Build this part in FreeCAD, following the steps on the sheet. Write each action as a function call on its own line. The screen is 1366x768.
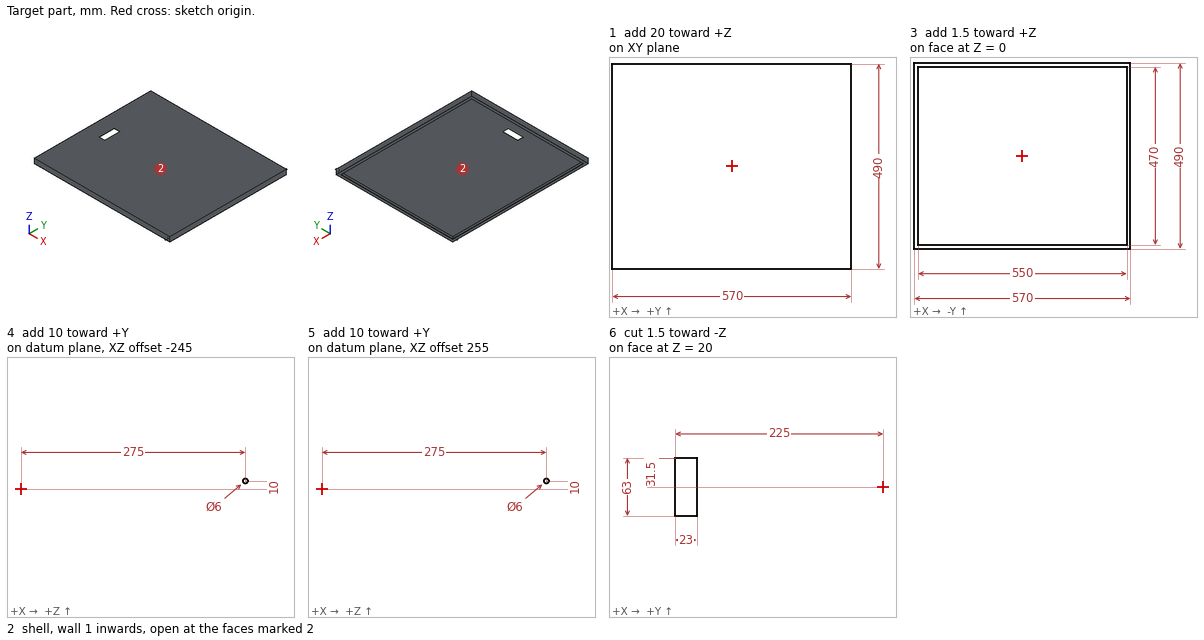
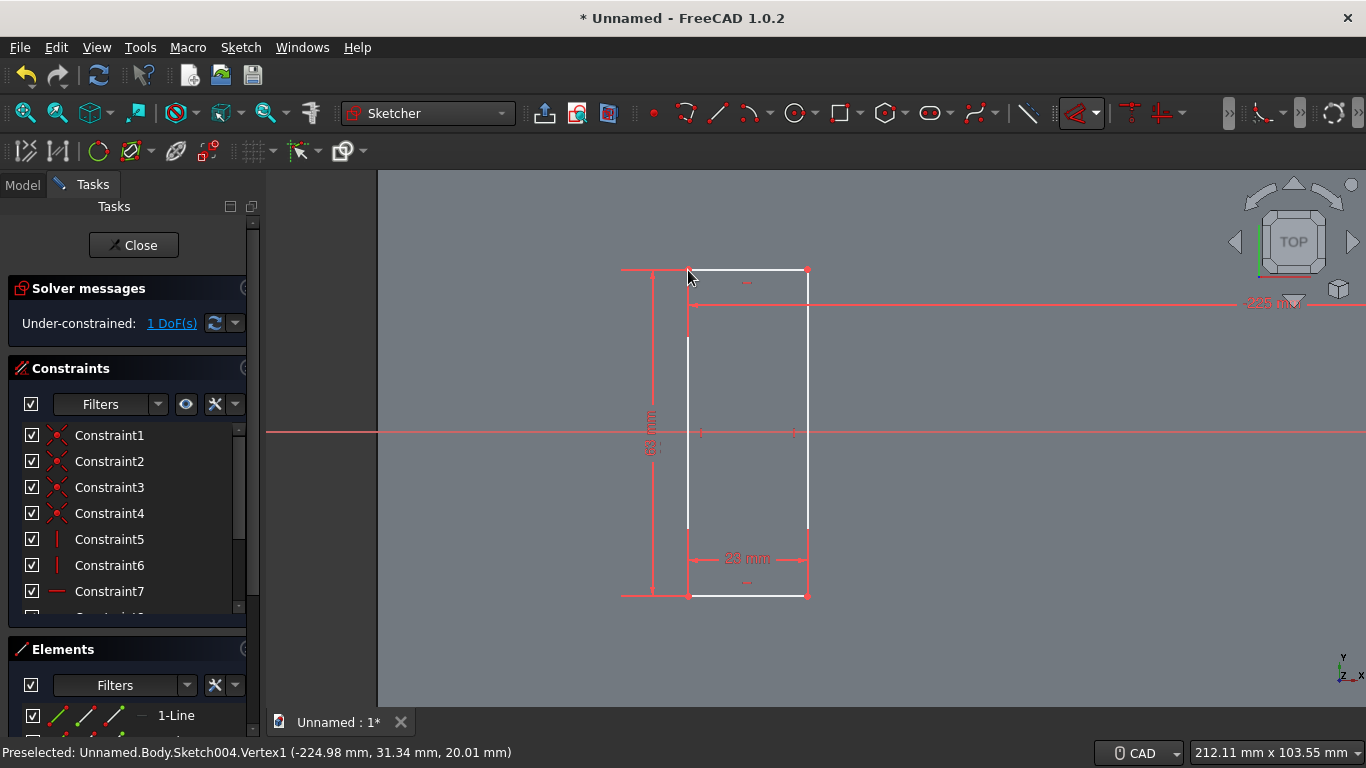
click(688, 270)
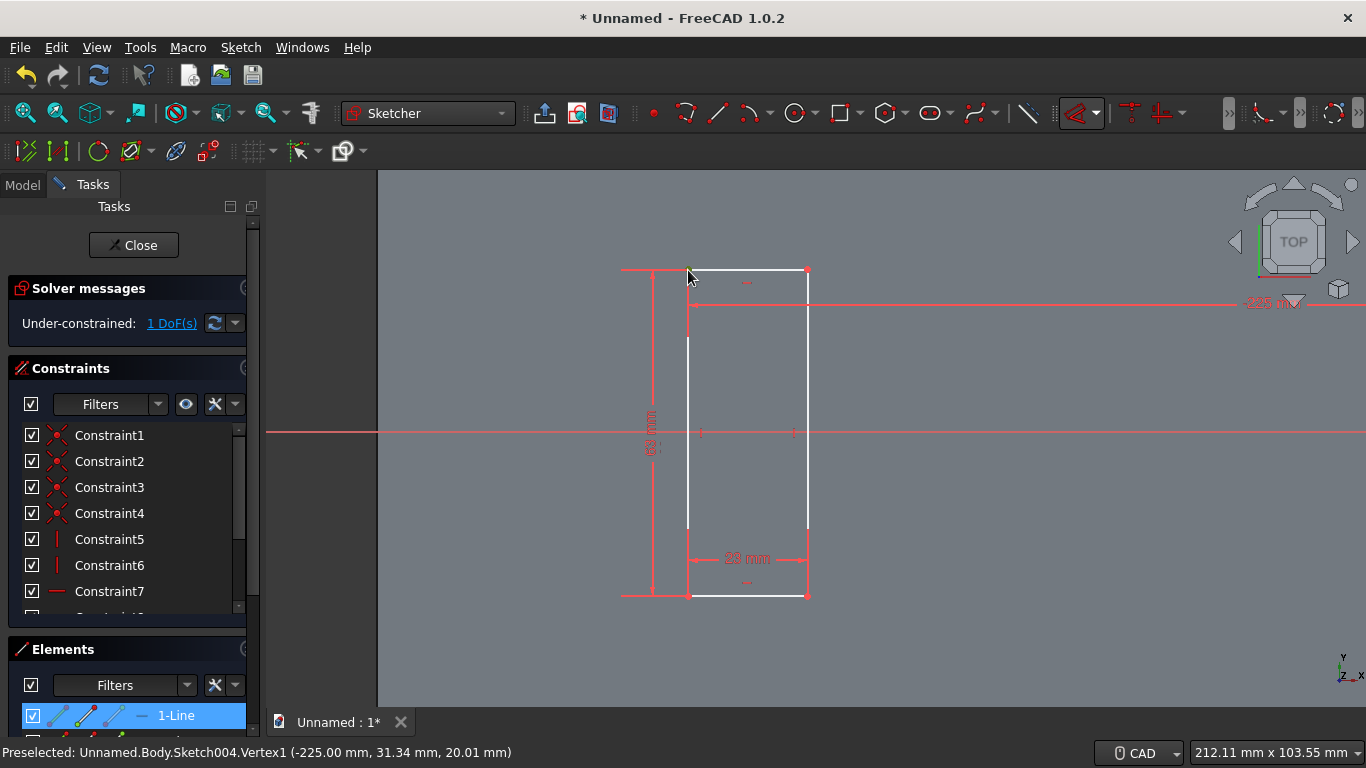
click(1098, 114)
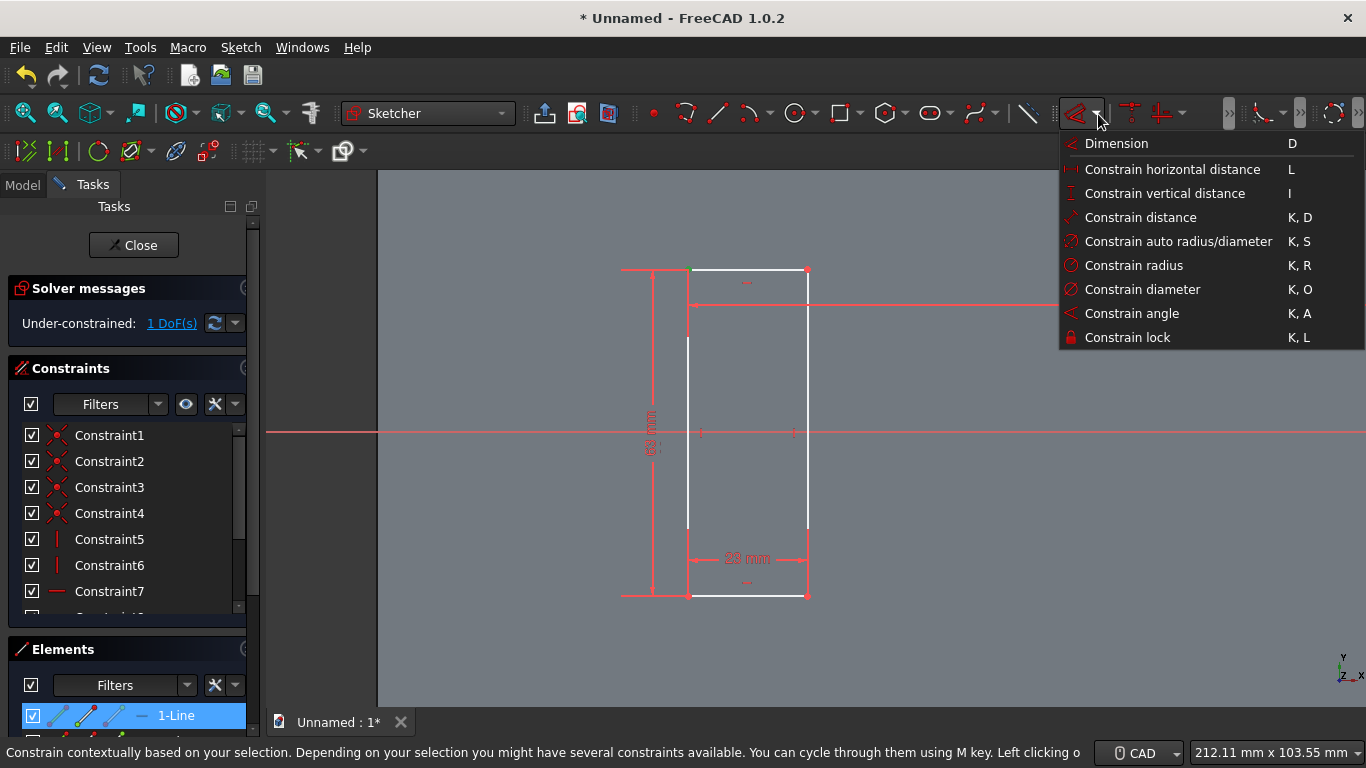
click(1212, 193)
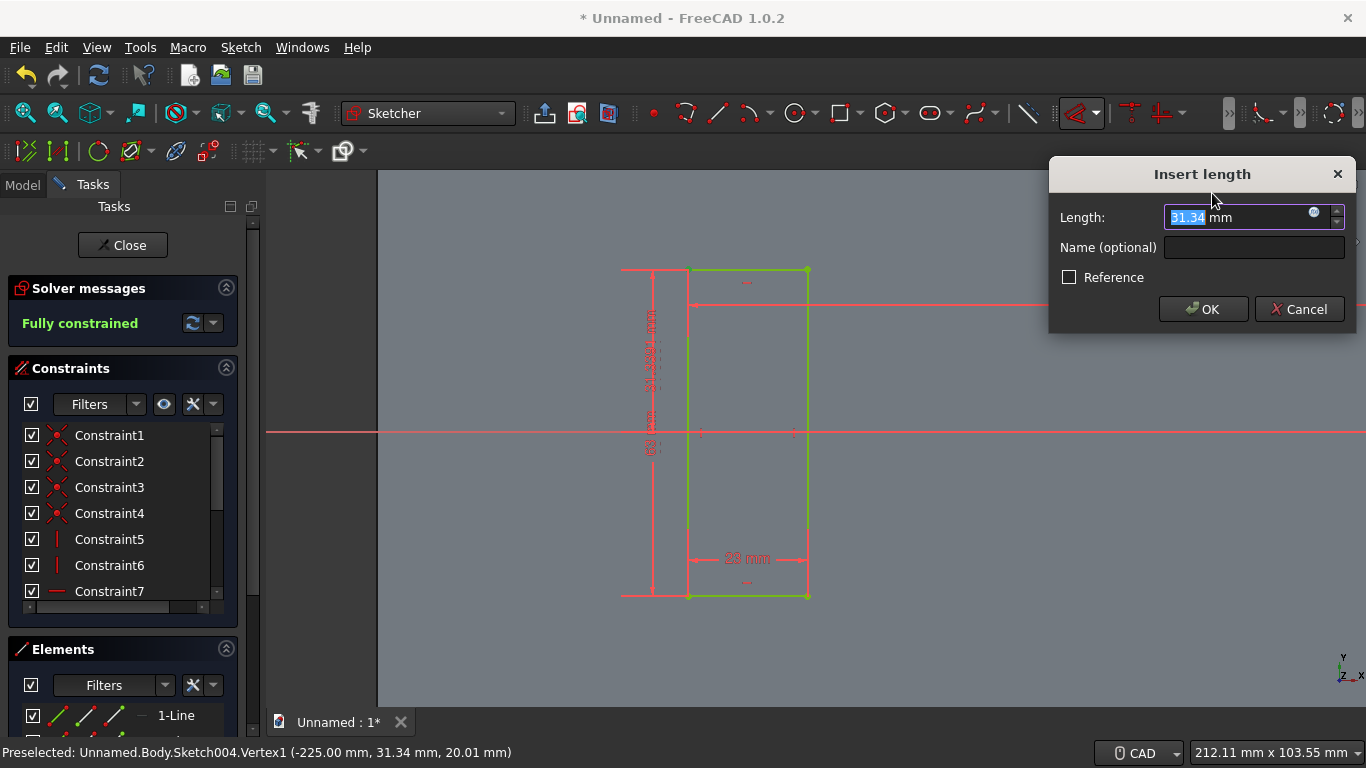
text(31.5)
key(Return)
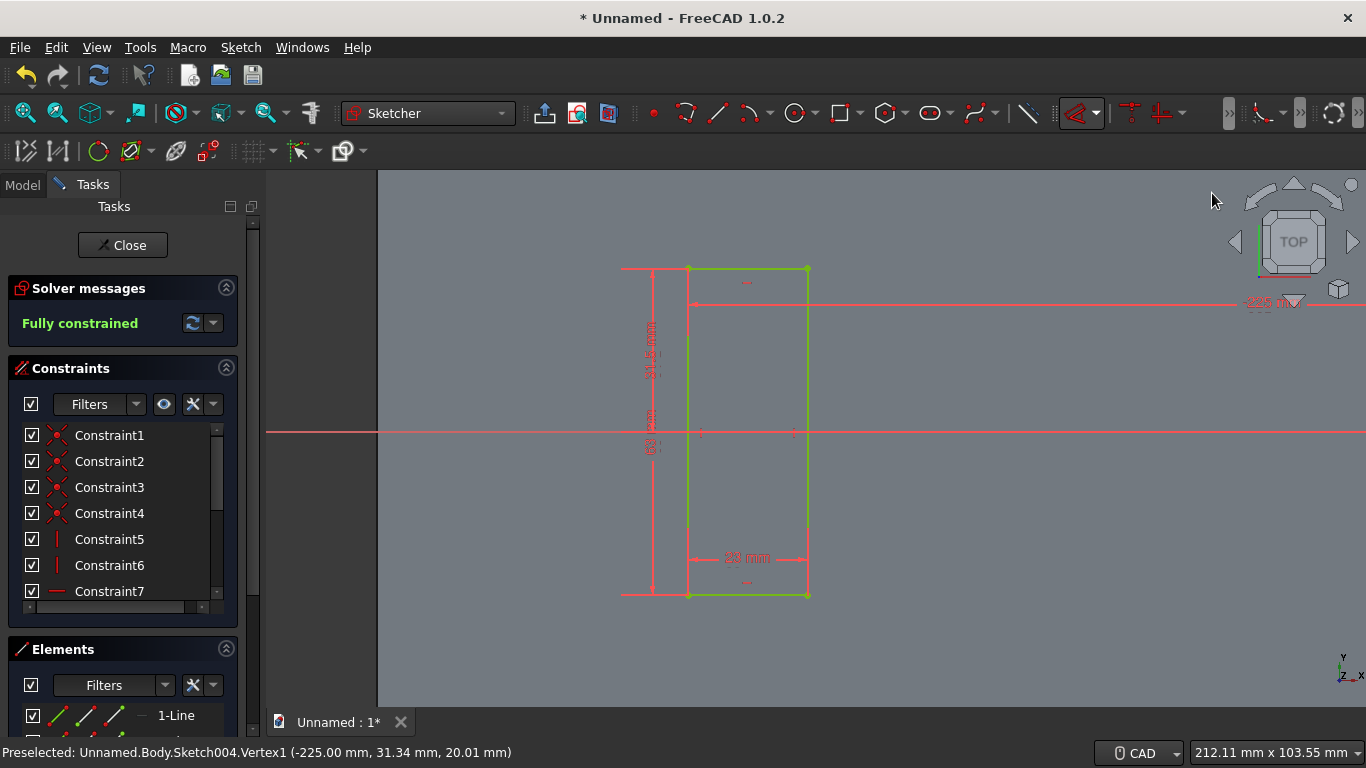
click(123, 245)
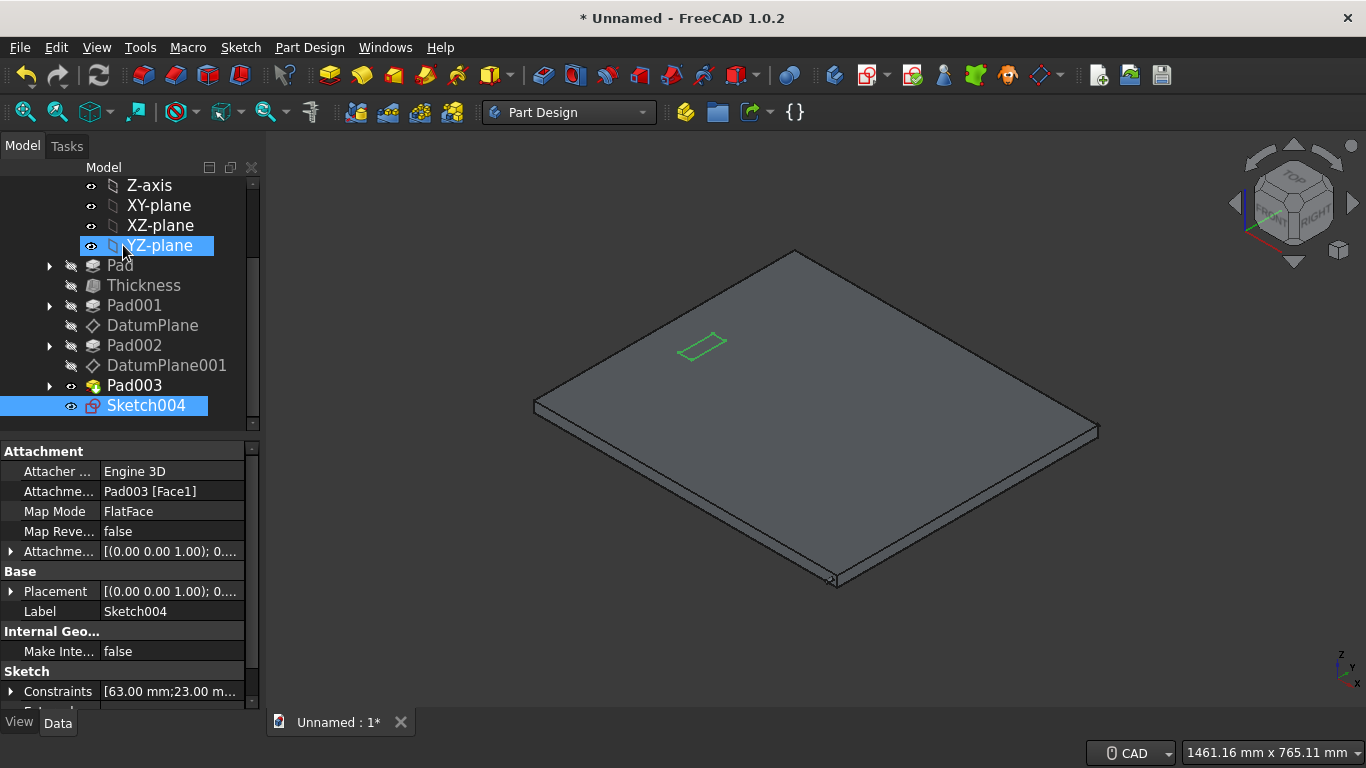
click(544, 76)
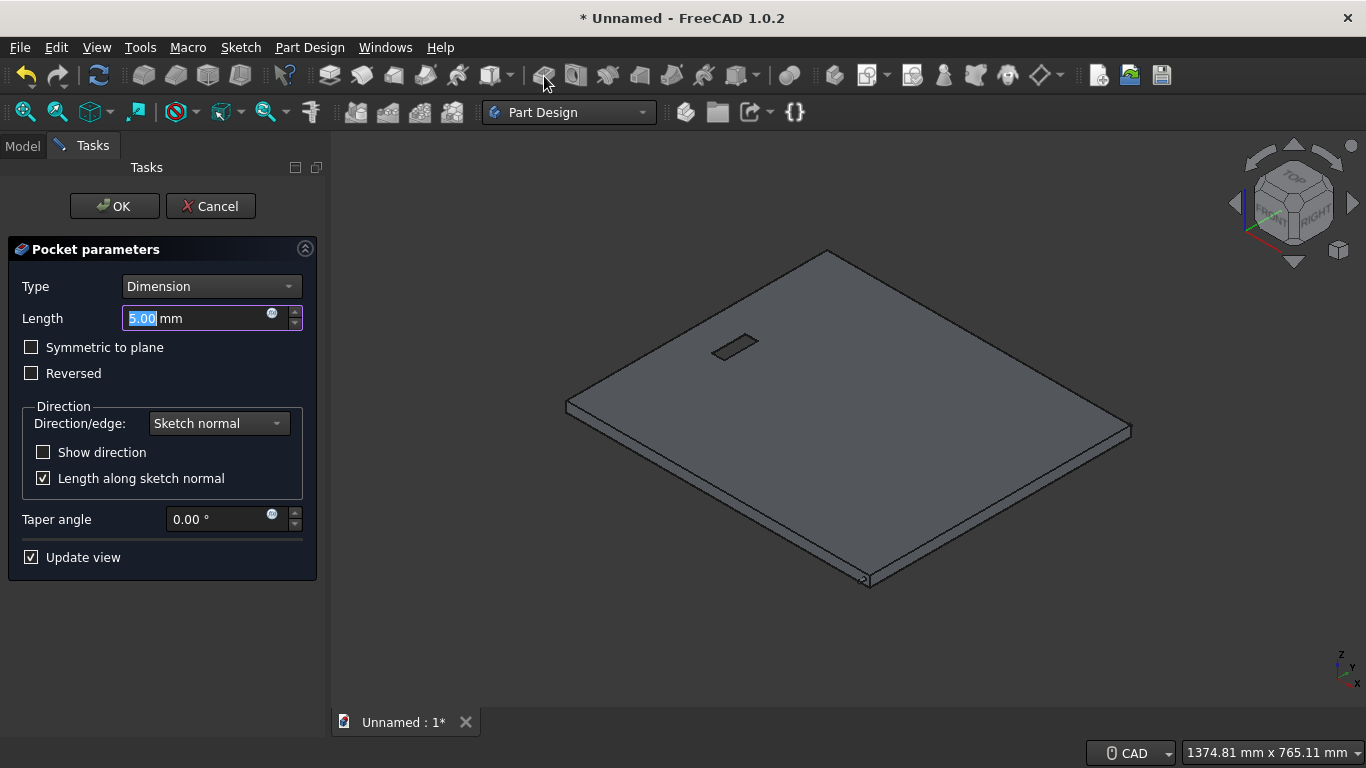
text(1.5)
key(Tab)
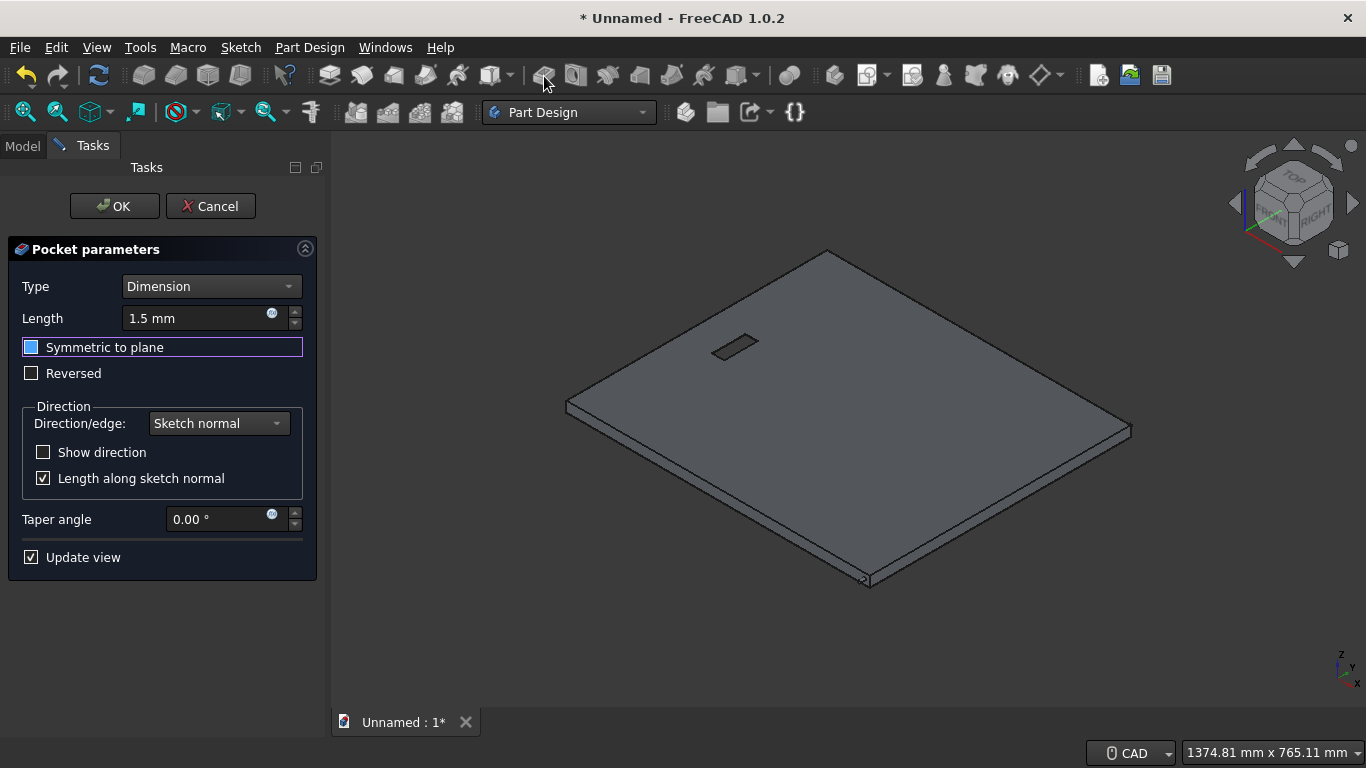
click(115, 206)